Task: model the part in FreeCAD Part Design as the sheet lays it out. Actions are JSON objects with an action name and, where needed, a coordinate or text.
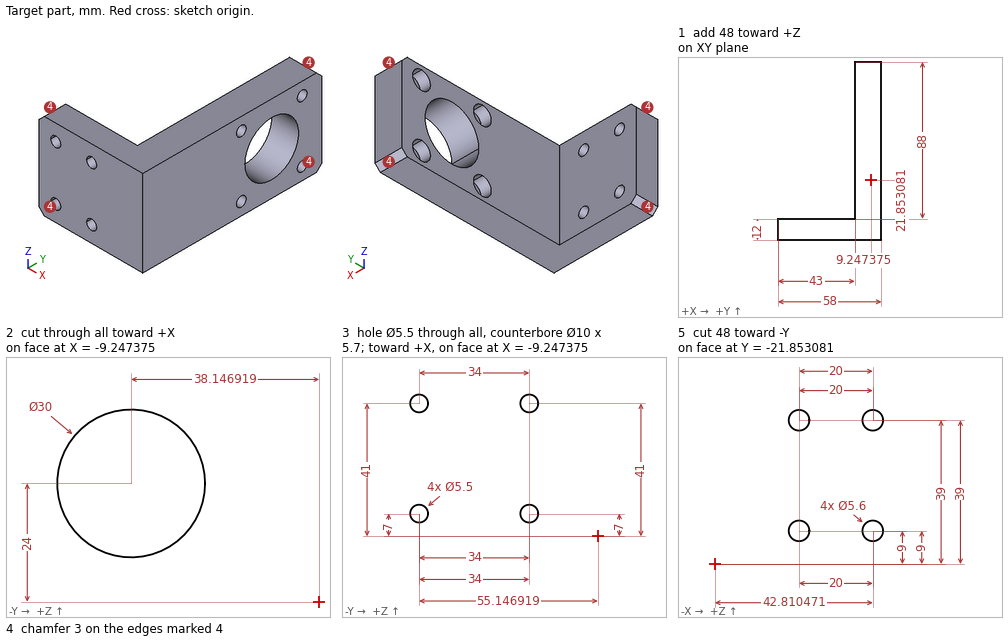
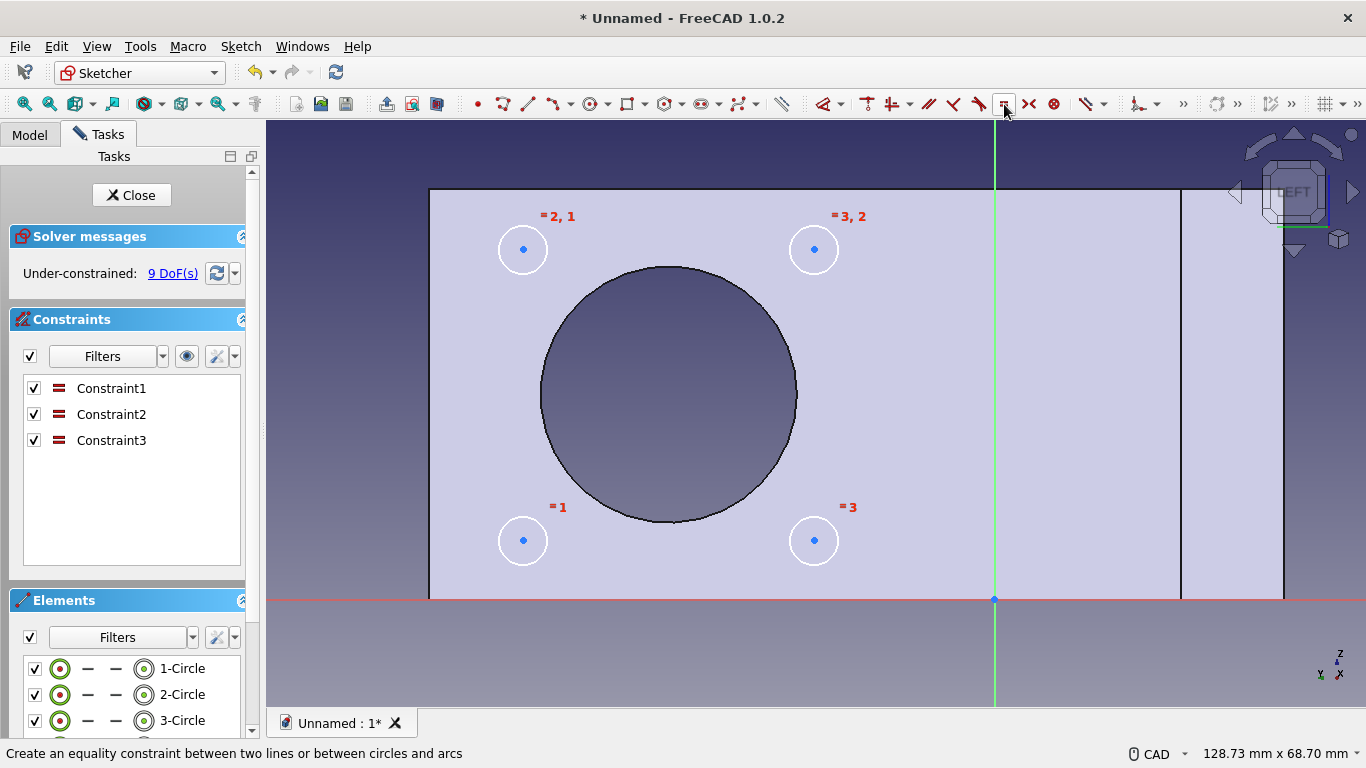
{"action": "left_click", "coordinate": [822, 104]}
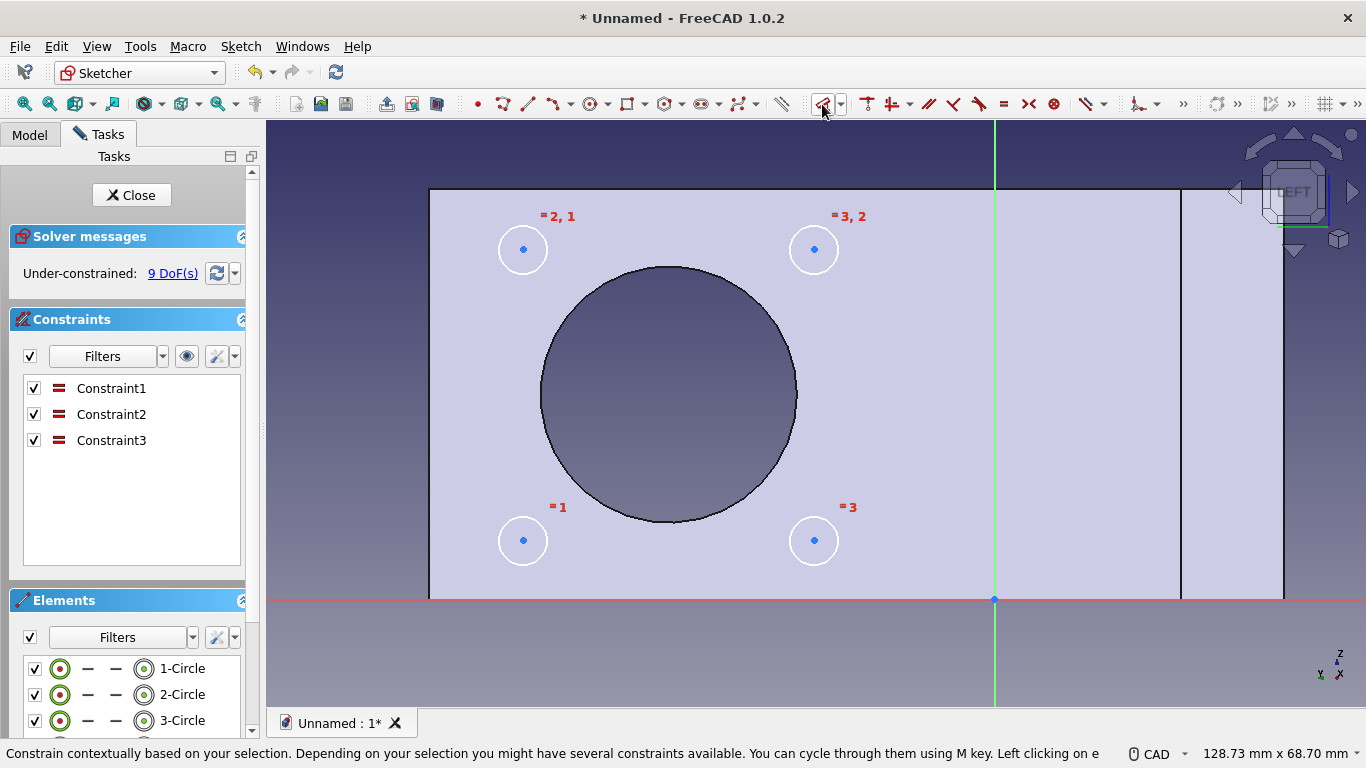
{"action": "left_click", "coordinate": [540, 524]}
{"action": "left_click", "coordinate": [563, 501]}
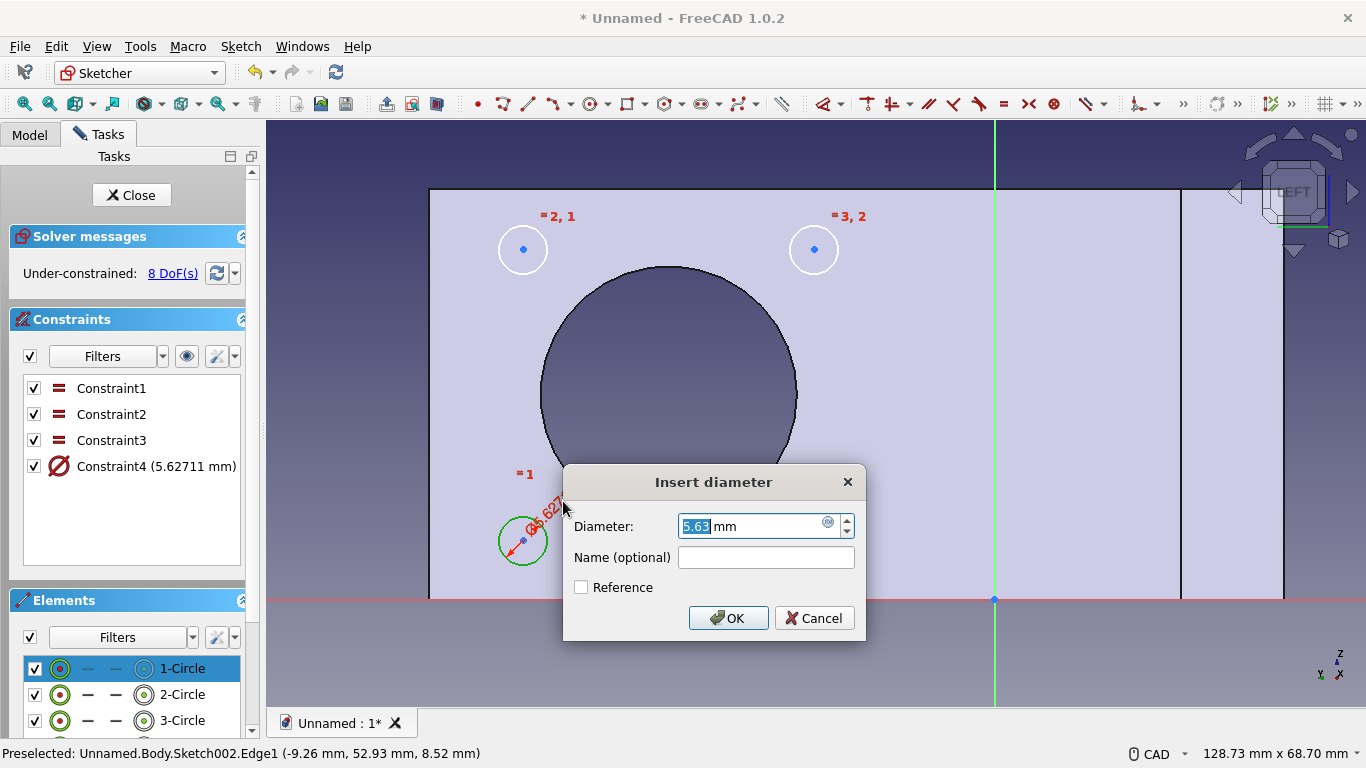
{"action": "type", "text": "5.5"}
{"action": "key", "text": "Return"}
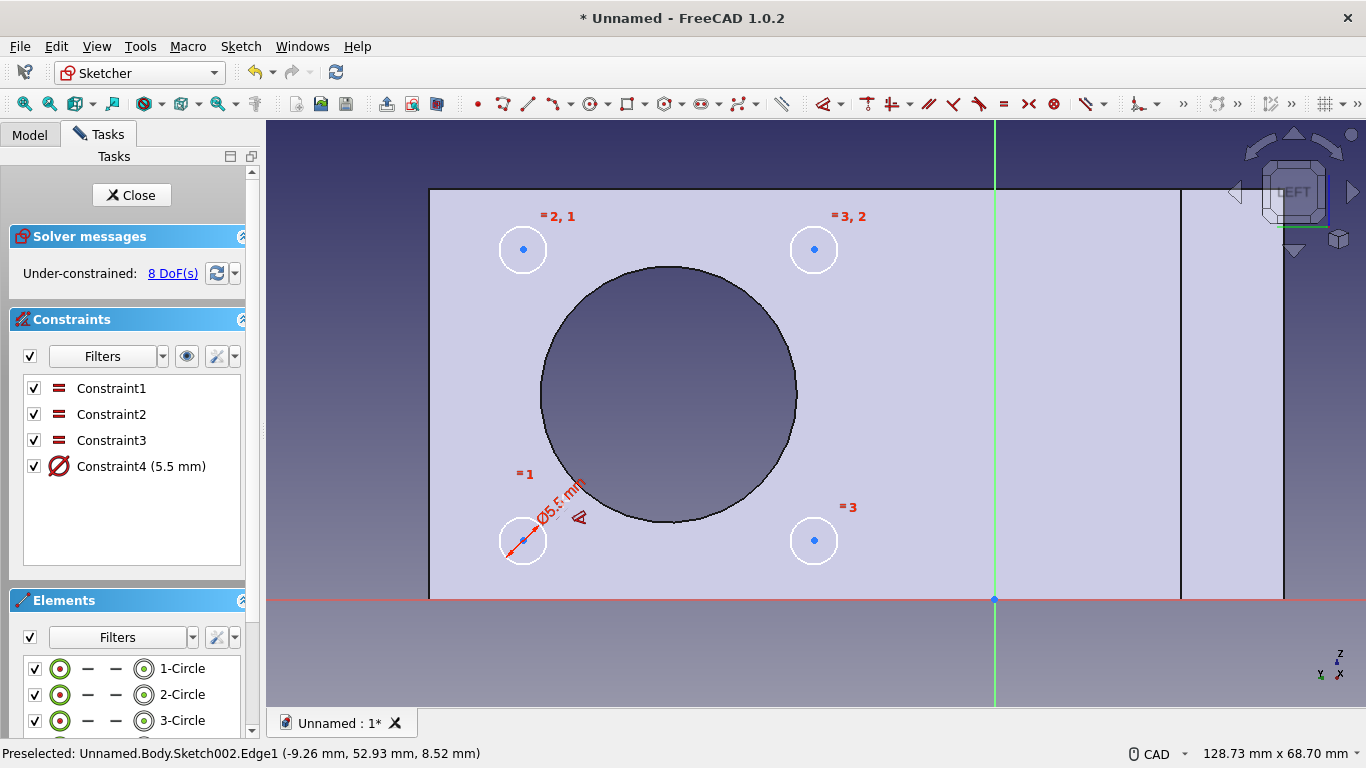
{"action": "left_click", "coordinate": [523, 541]}
{"action": "left_click", "coordinate": [1029, 570]}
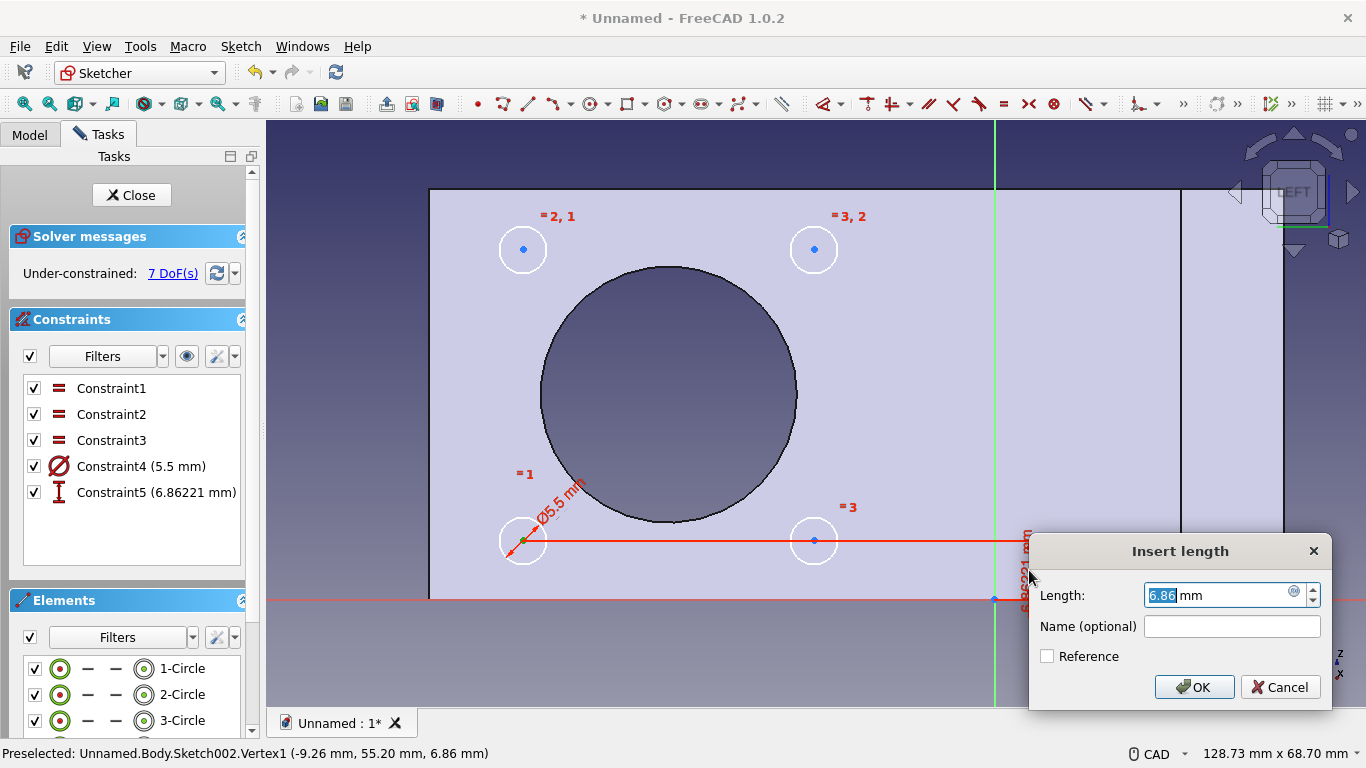
{"action": "type", "text": "7"}
{"action": "key", "text": "Return"}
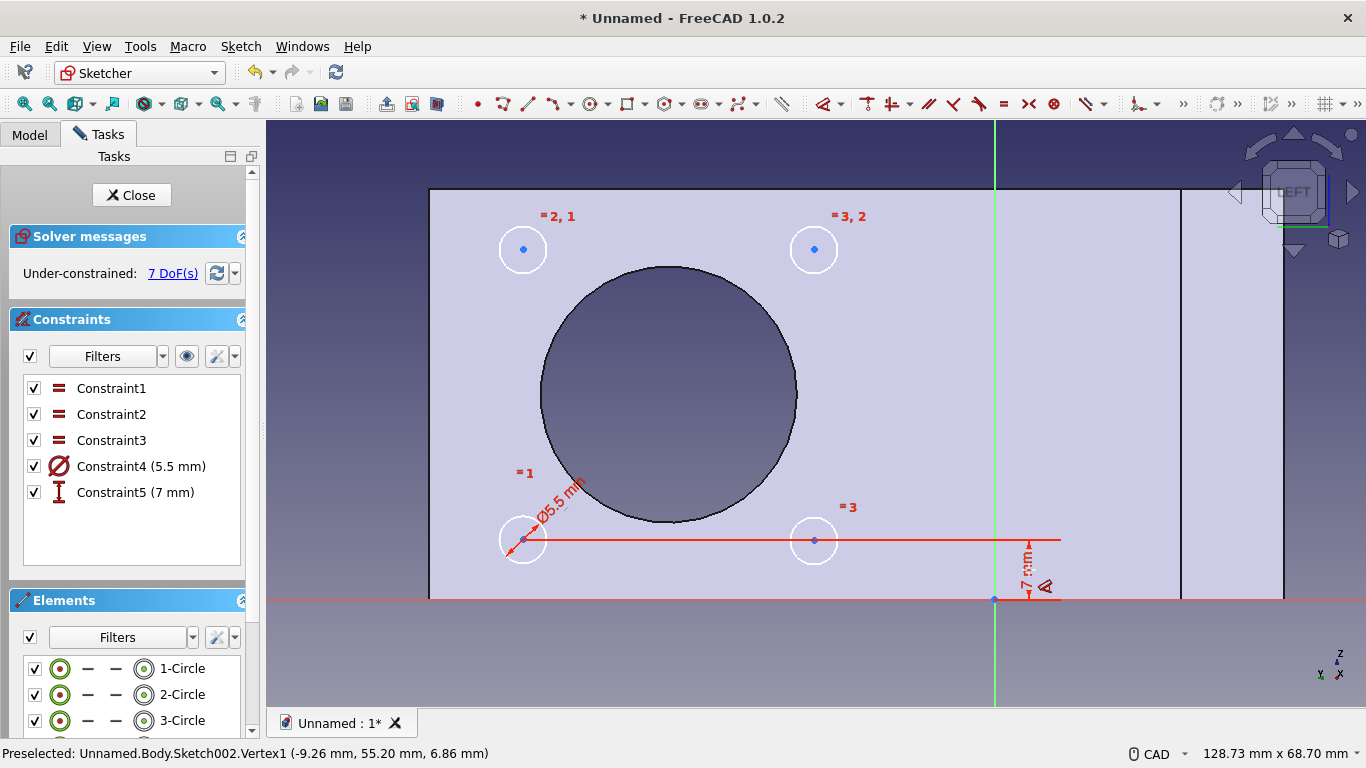
{"action": "left_click", "coordinate": [814, 541]}
{"action": "left_click", "coordinate": [1029, 550]}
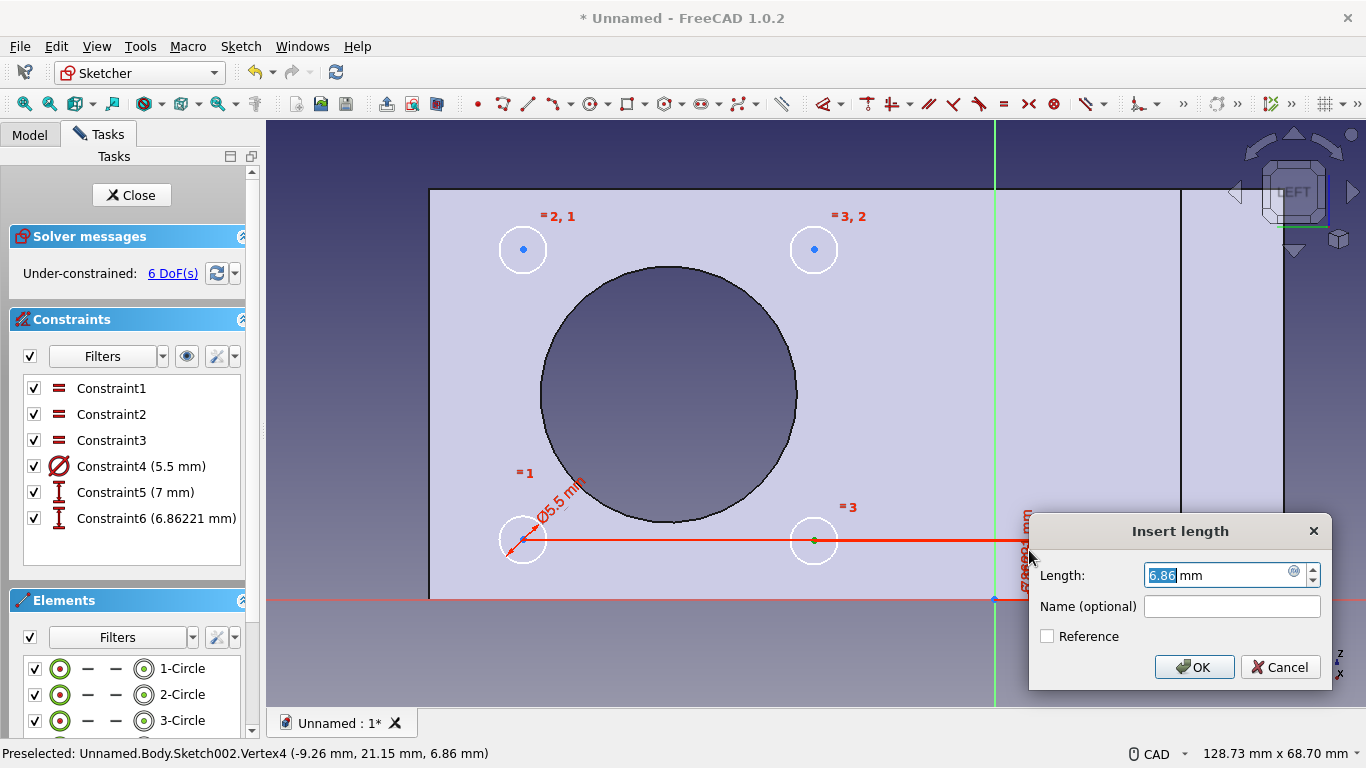
{"action": "type", "text": "7"}
{"action": "key", "text": "Return"}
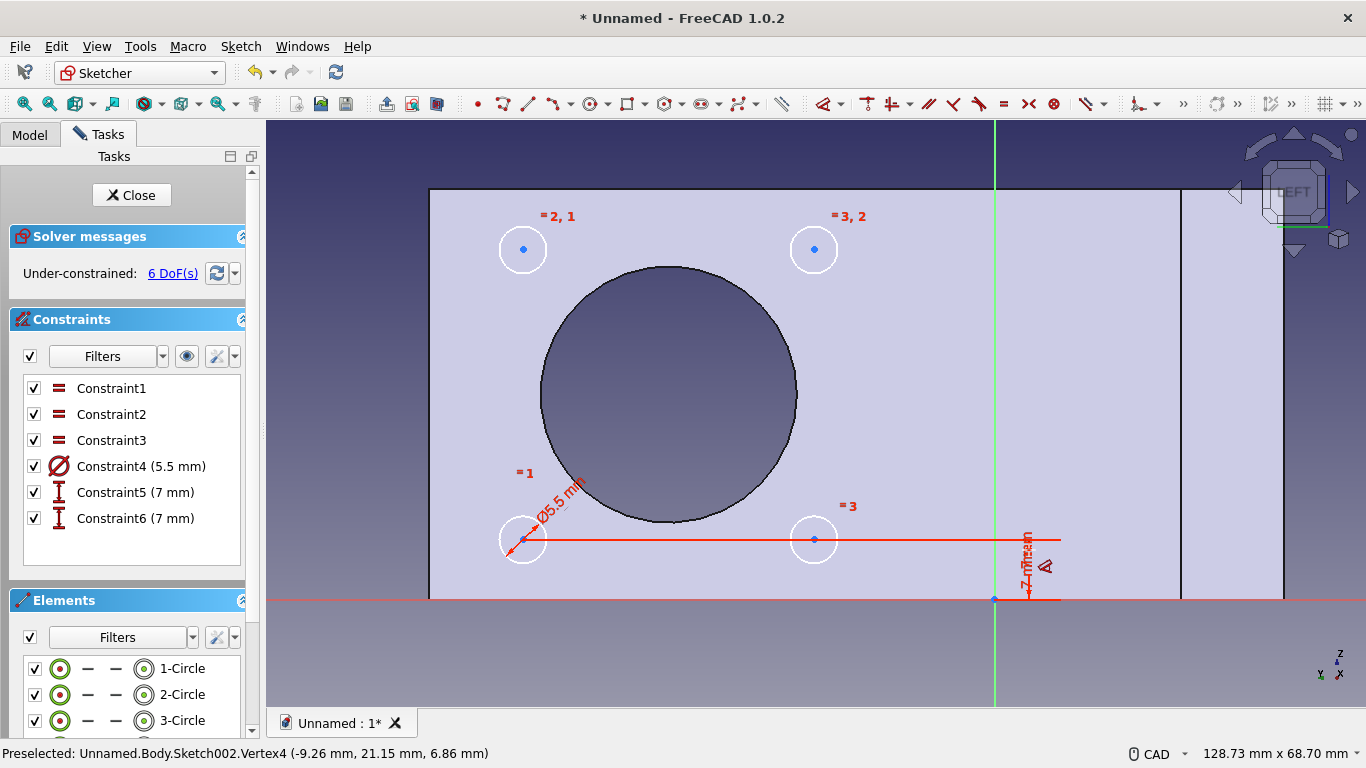
{"action": "left_click", "coordinate": [523, 250]}
{"action": "left_click", "coordinate": [1029, 425]}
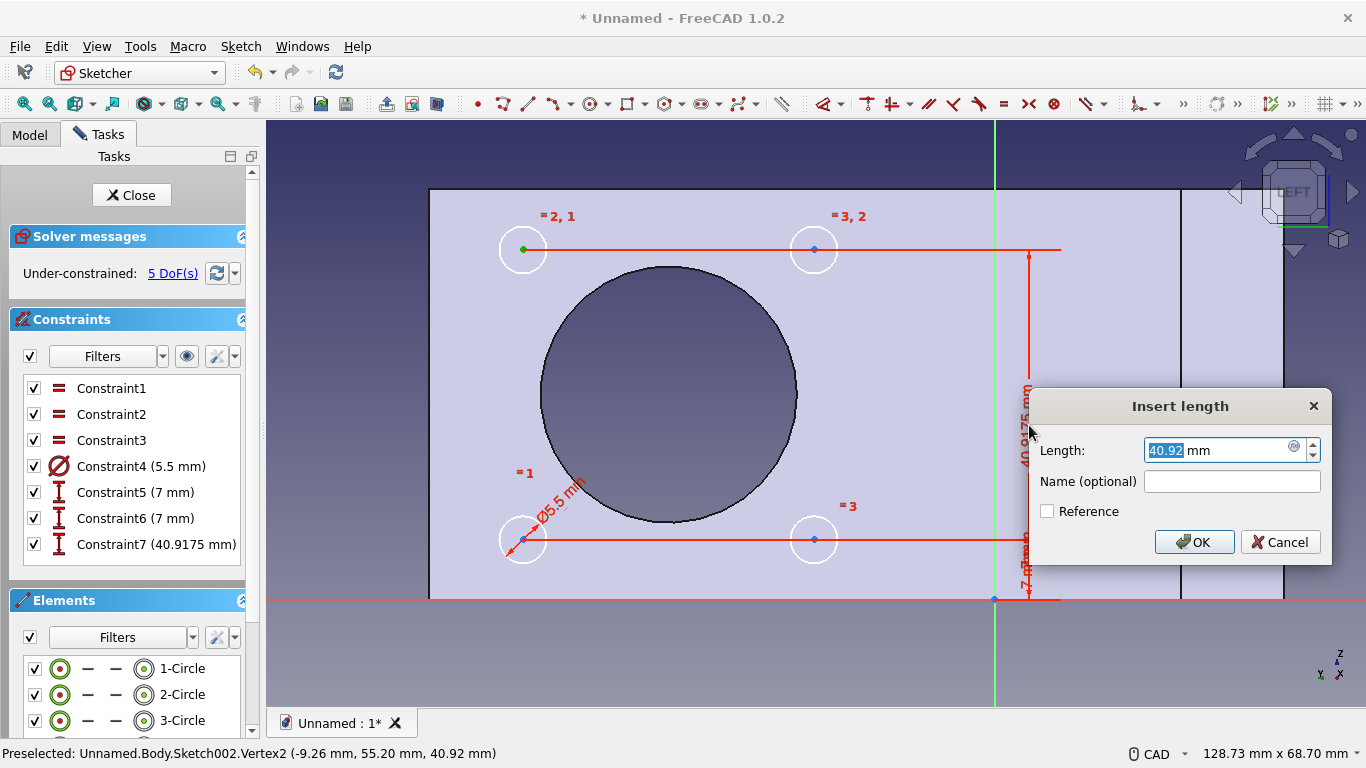
{"action": "type", "text": "41"}
{"action": "key", "text": "Return"}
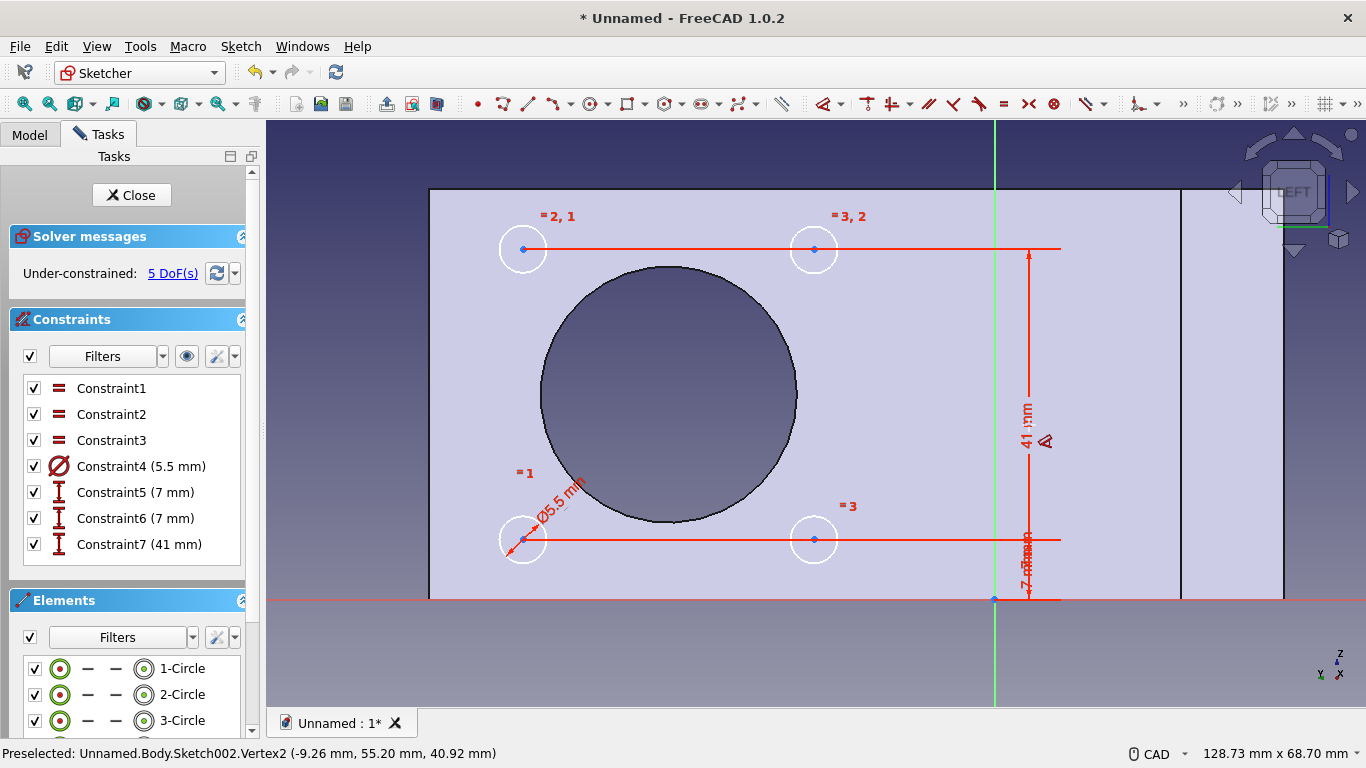
{"action": "left_click", "coordinate": [814, 250]}
{"action": "left_click", "coordinate": [1029, 344]}